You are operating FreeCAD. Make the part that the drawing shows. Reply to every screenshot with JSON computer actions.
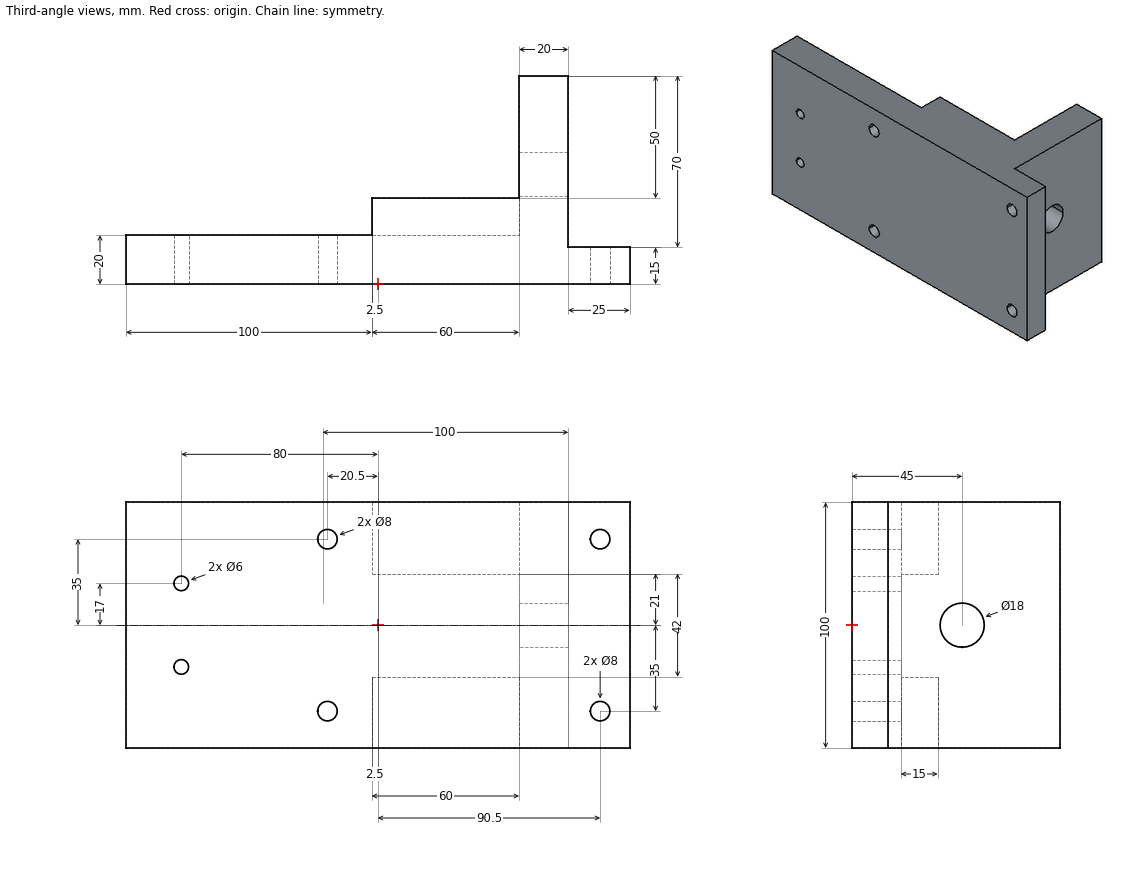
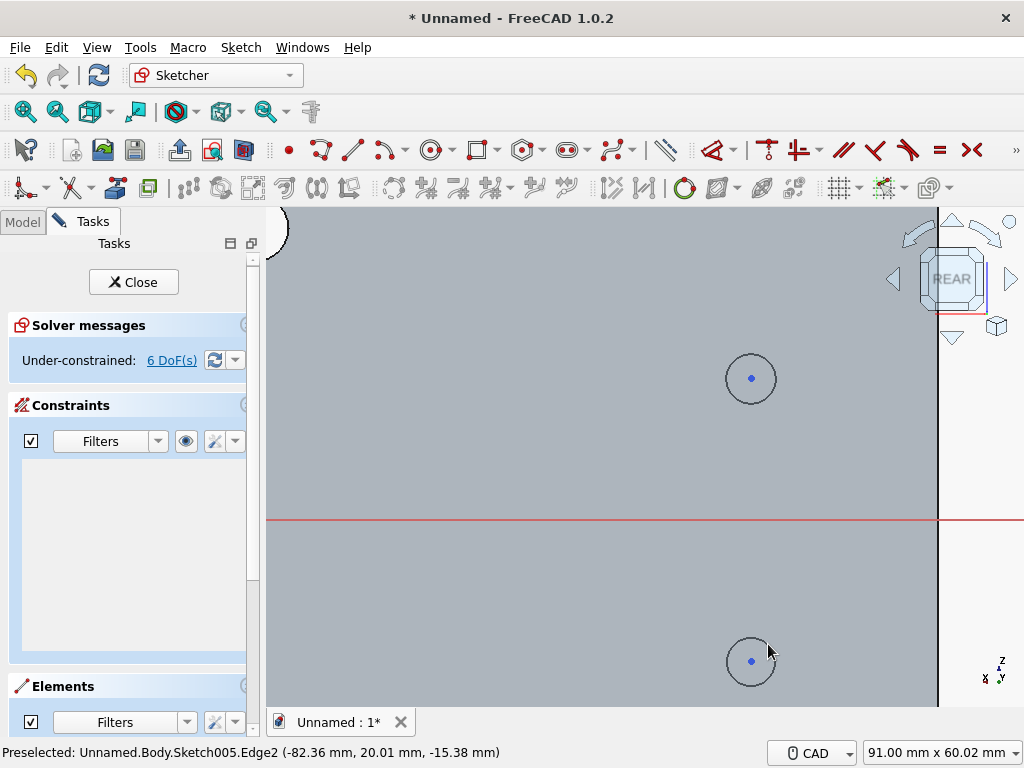
{"action": "left_click", "coordinate": [768, 361]}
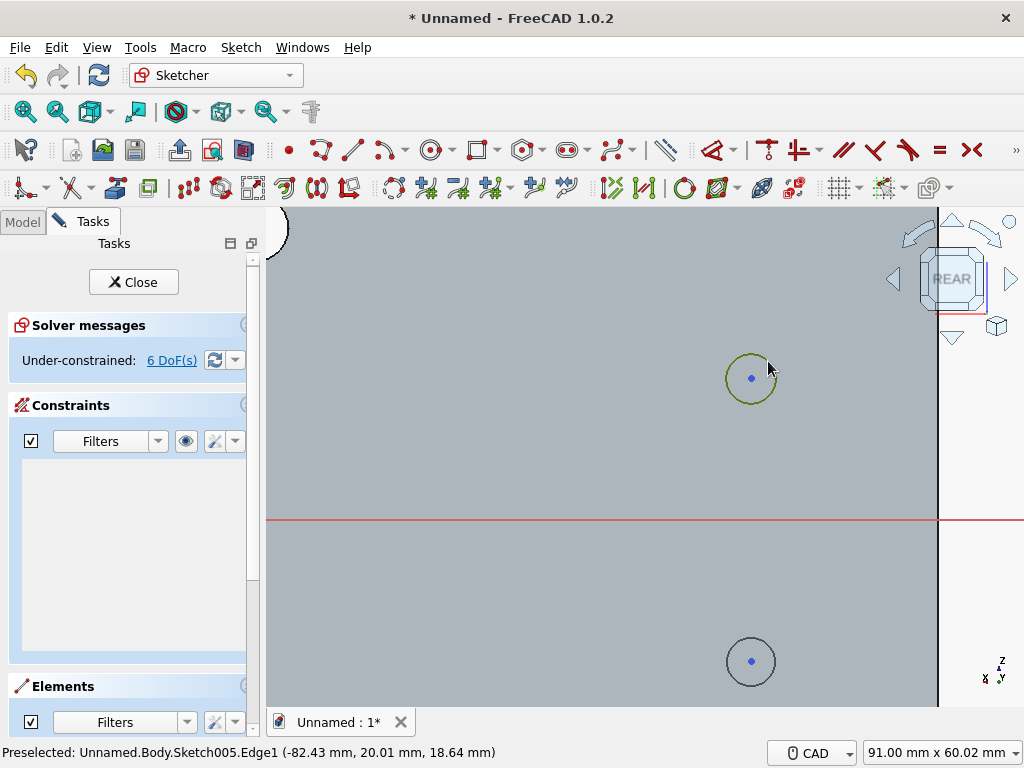
{"action": "left_click", "coordinate": [768, 645]}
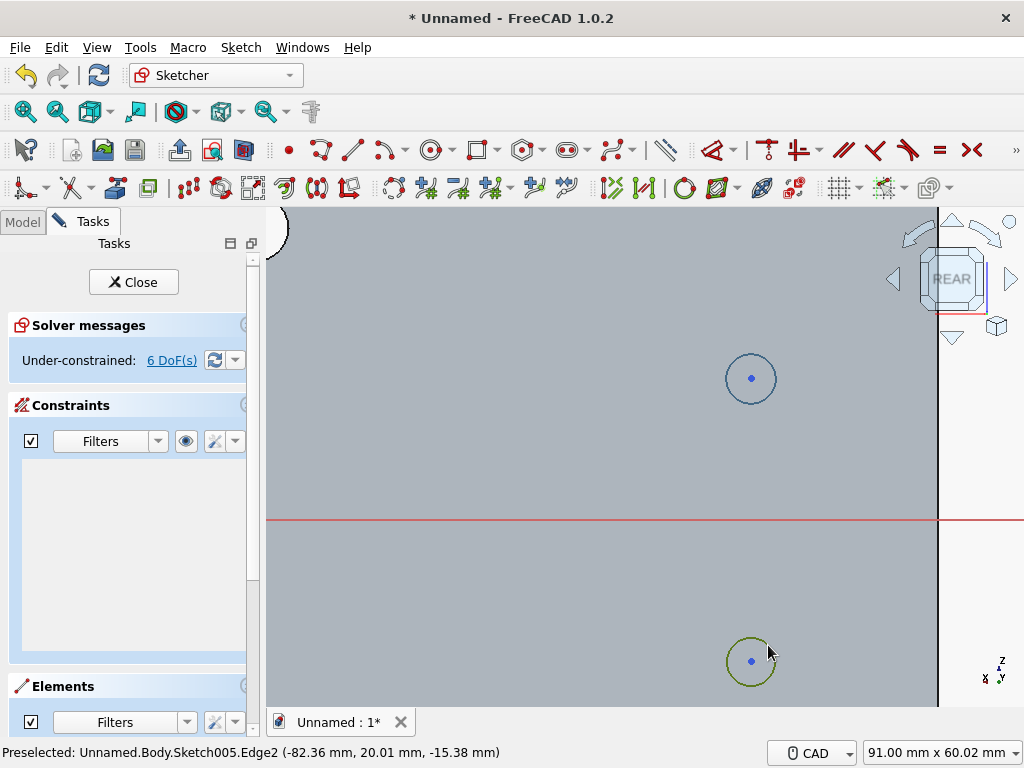
{"action": "left_click", "coordinate": [940, 150]}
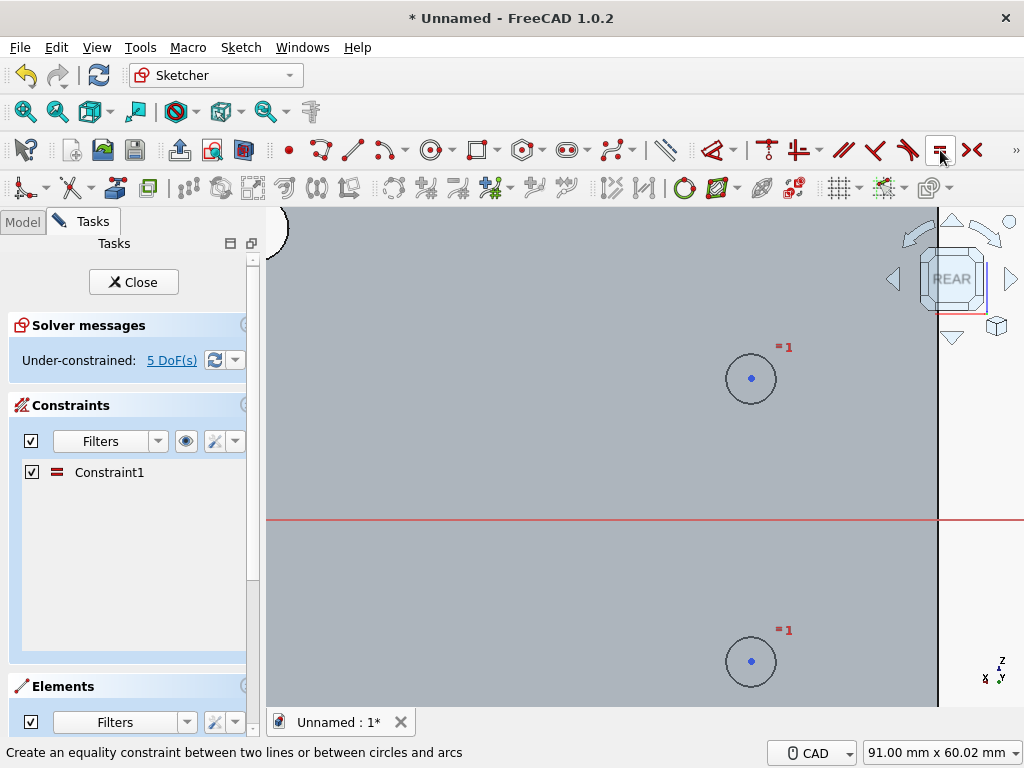
{"action": "left_click", "coordinate": [751, 379]}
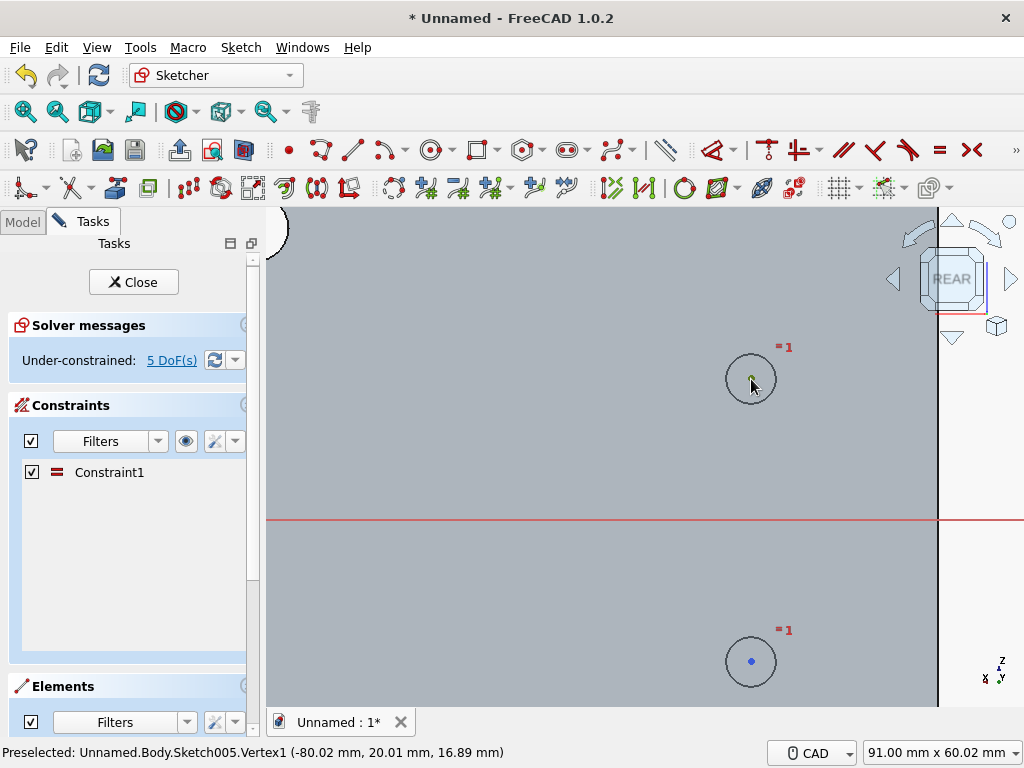
{"action": "left_click", "coordinate": [751, 662]}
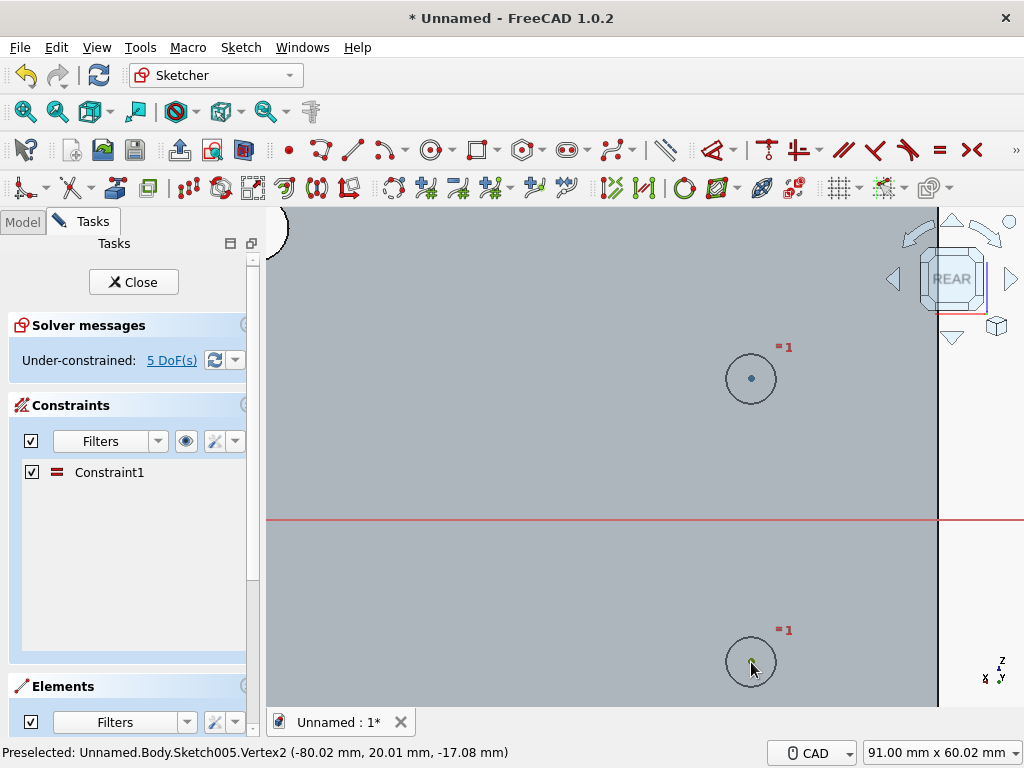
{"action": "left_click", "coordinate": [334, 520]}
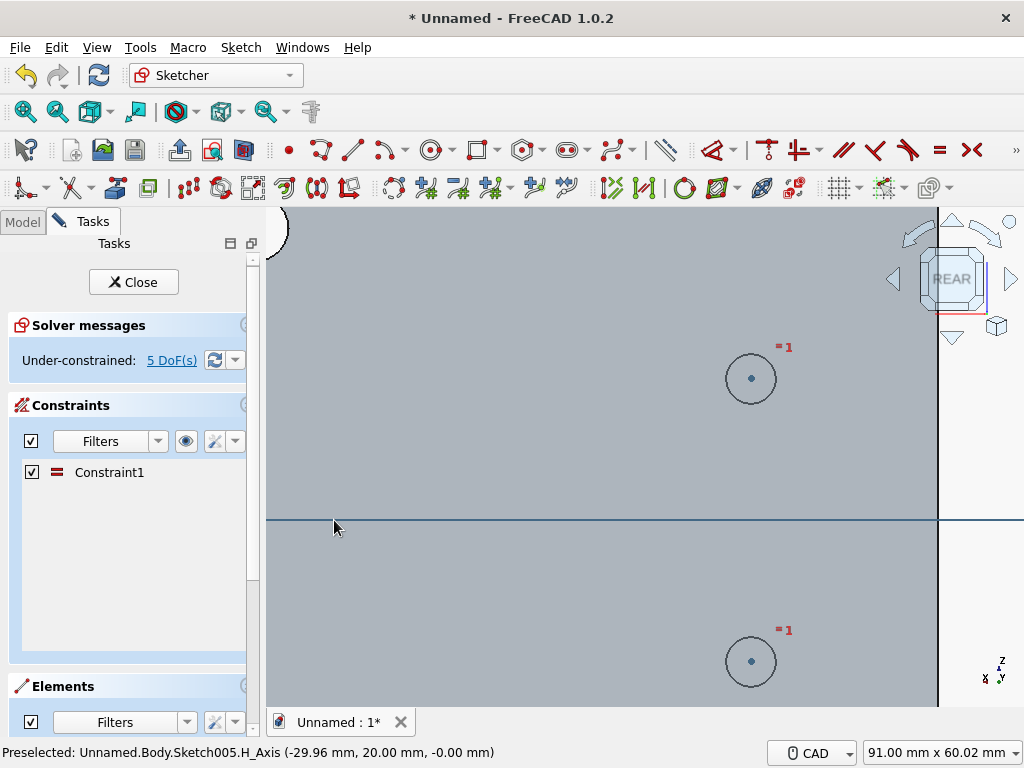
{"action": "left_click", "coordinate": [972, 150]}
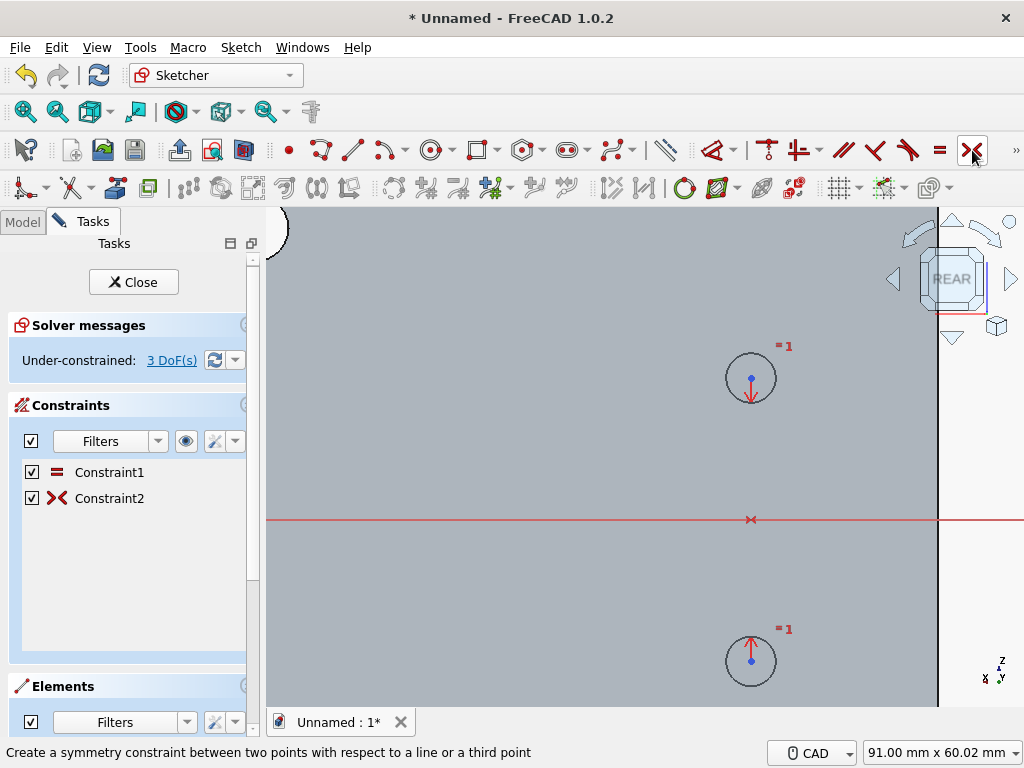
{"action": "left_click", "coordinate": [712, 150]}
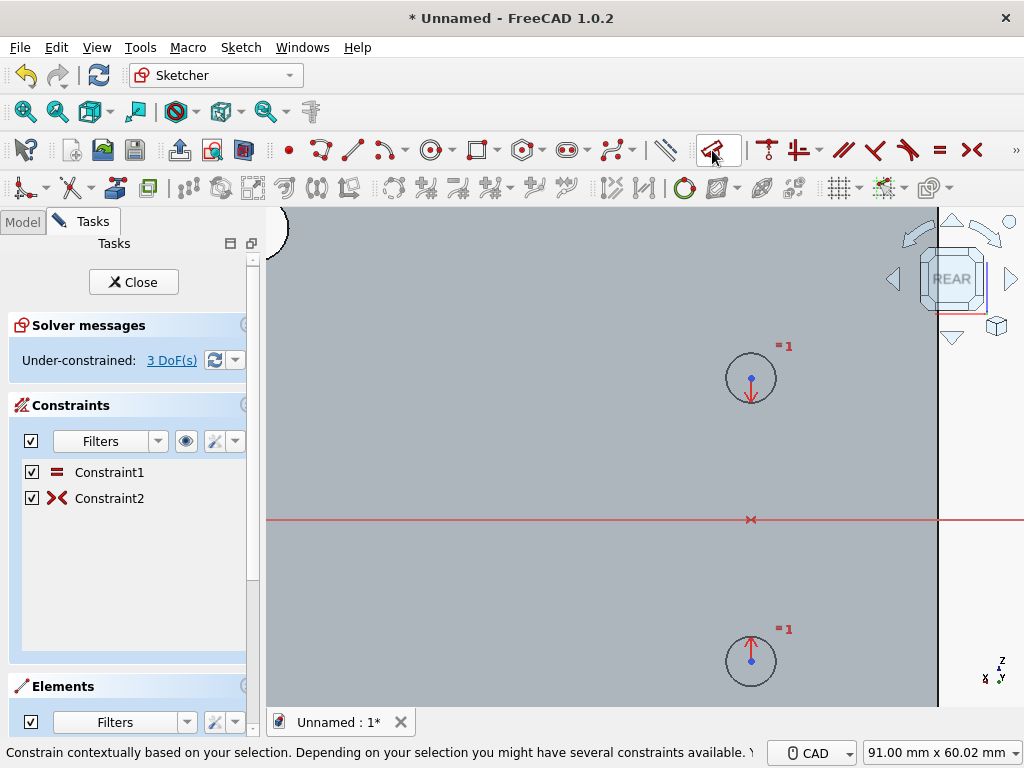
{"action": "left_click", "coordinate": [768, 360]}
{"action": "left_click", "coordinate": [790, 337]}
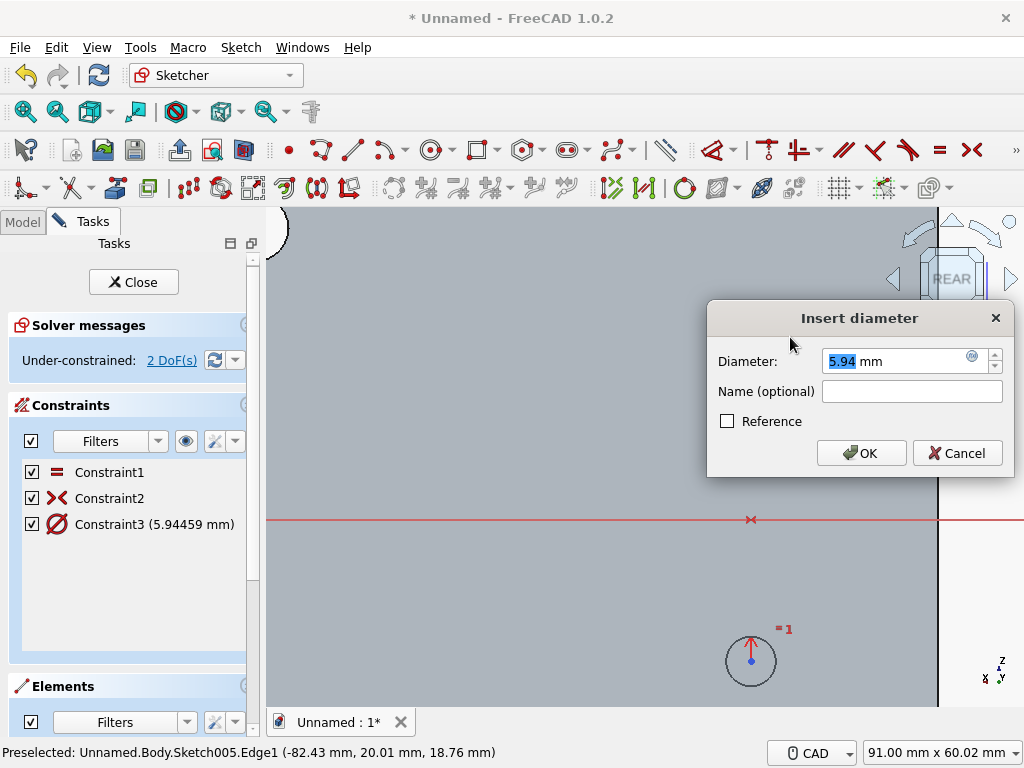
{"action": "type", "text": "6"}
{"action": "key", "text": "Return"}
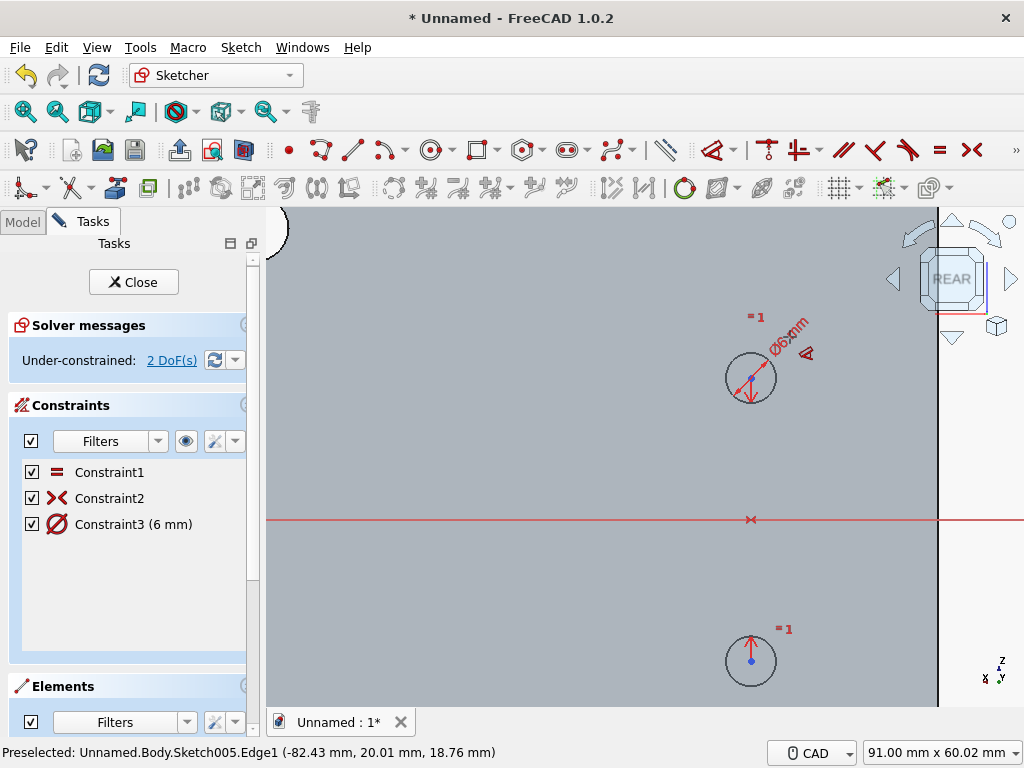
{"action": "left_click", "coordinate": [751, 378]}
{"action": "left_click", "coordinate": [523, 344]}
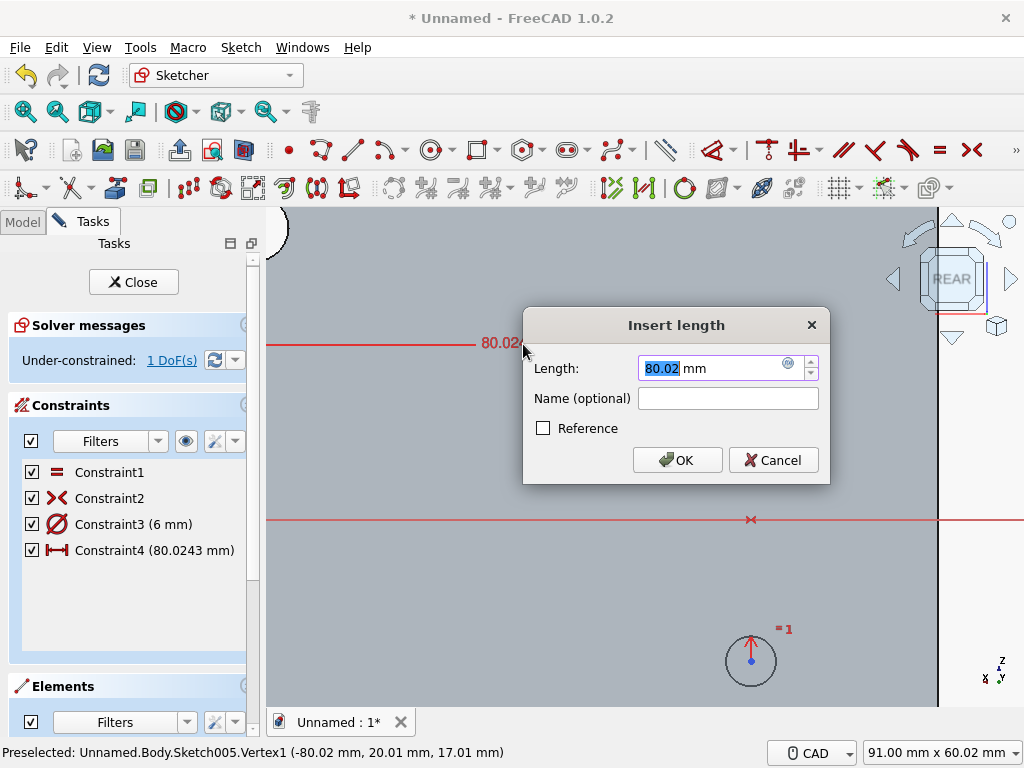
{"action": "type", "text": "80"}
{"action": "key", "text": "Return"}